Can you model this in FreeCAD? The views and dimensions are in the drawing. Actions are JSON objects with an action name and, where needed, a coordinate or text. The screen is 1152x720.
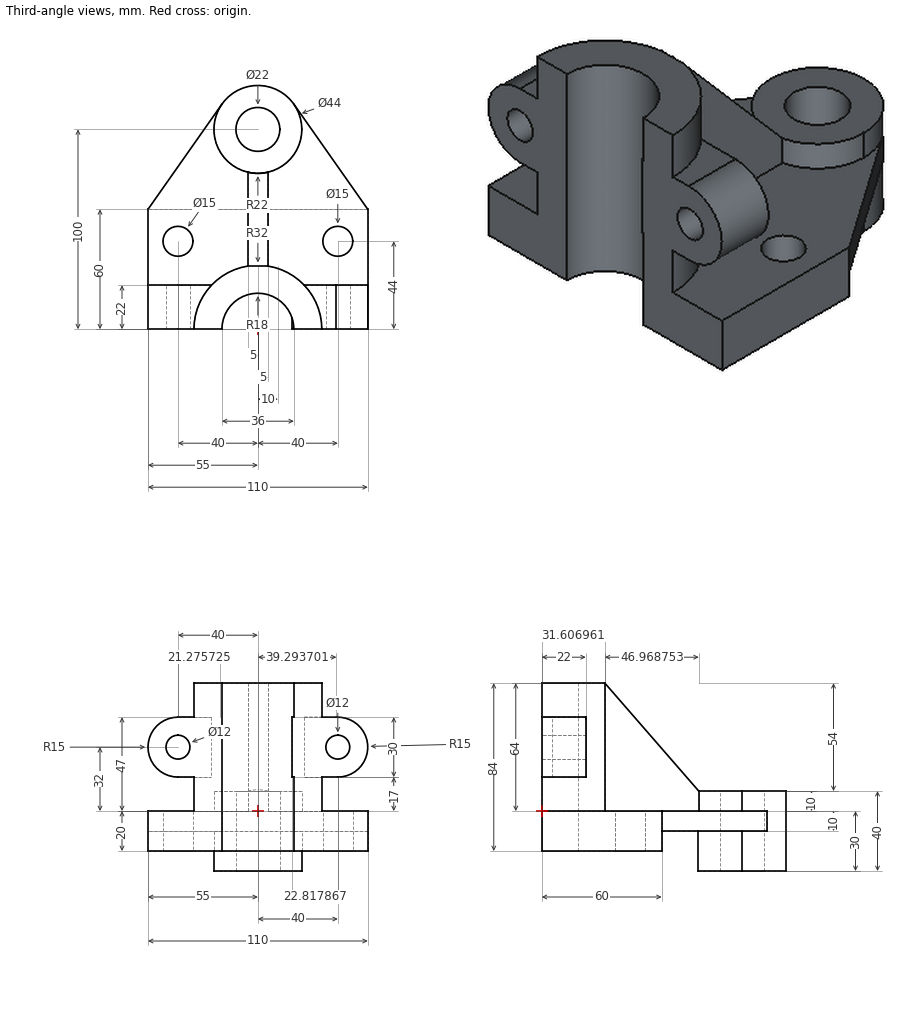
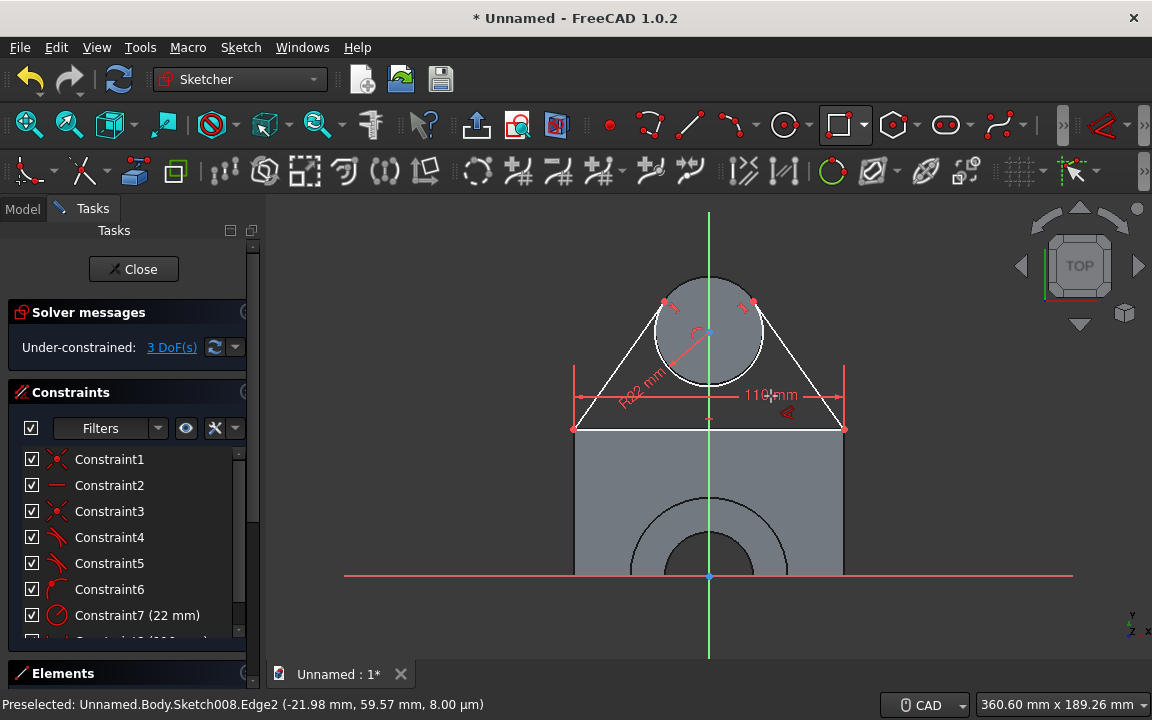
{"action": "left_click", "coordinate": [574, 430]}
{"action": "left_click", "coordinate": [641, 610]}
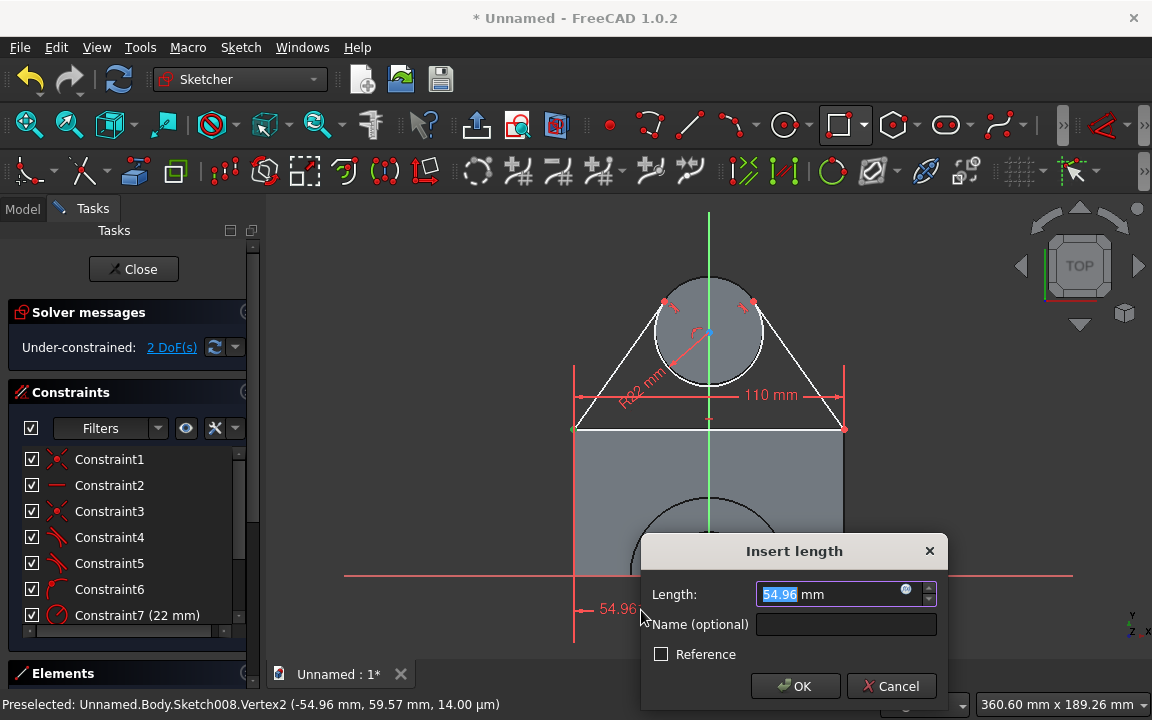
{"action": "type", "text": "55"}
{"action": "key", "text": "Return"}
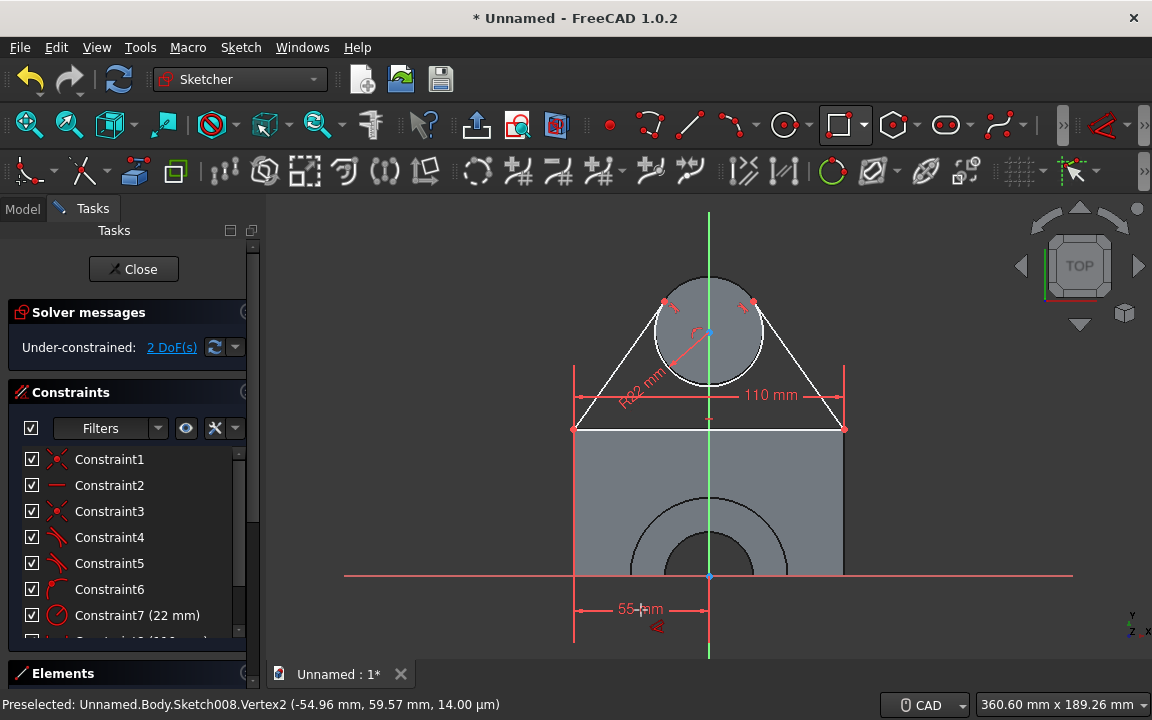
{"action": "left_click", "coordinate": [574, 430]}
{"action": "left_click", "coordinate": [540, 503]}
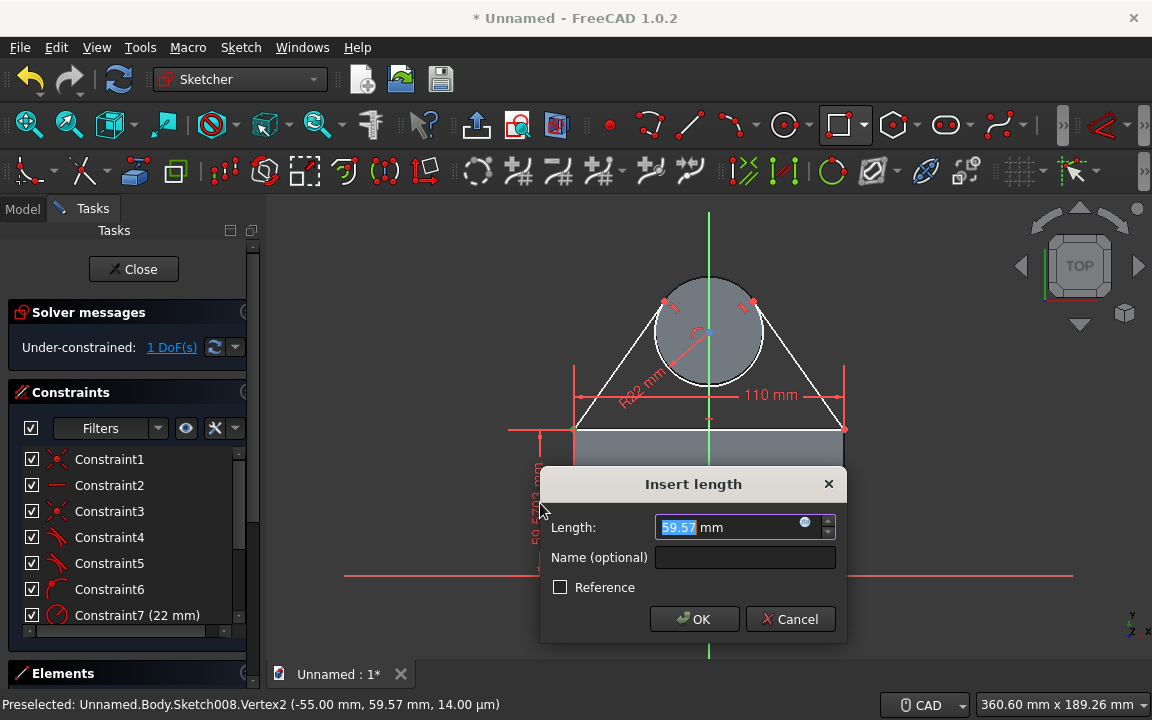
{"action": "type", "text": "60"}
{"action": "key", "text": "Return"}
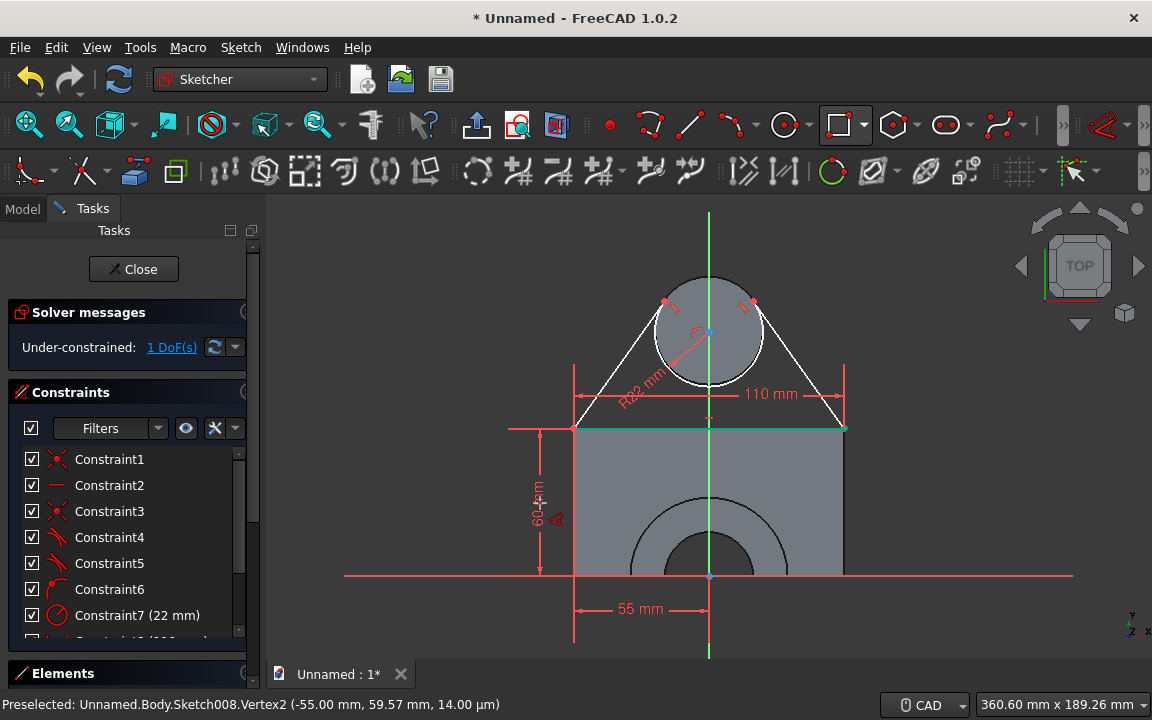
{"action": "left_click", "coordinate": [709, 333]}
{"action": "left_click", "coordinate": [743, 454]}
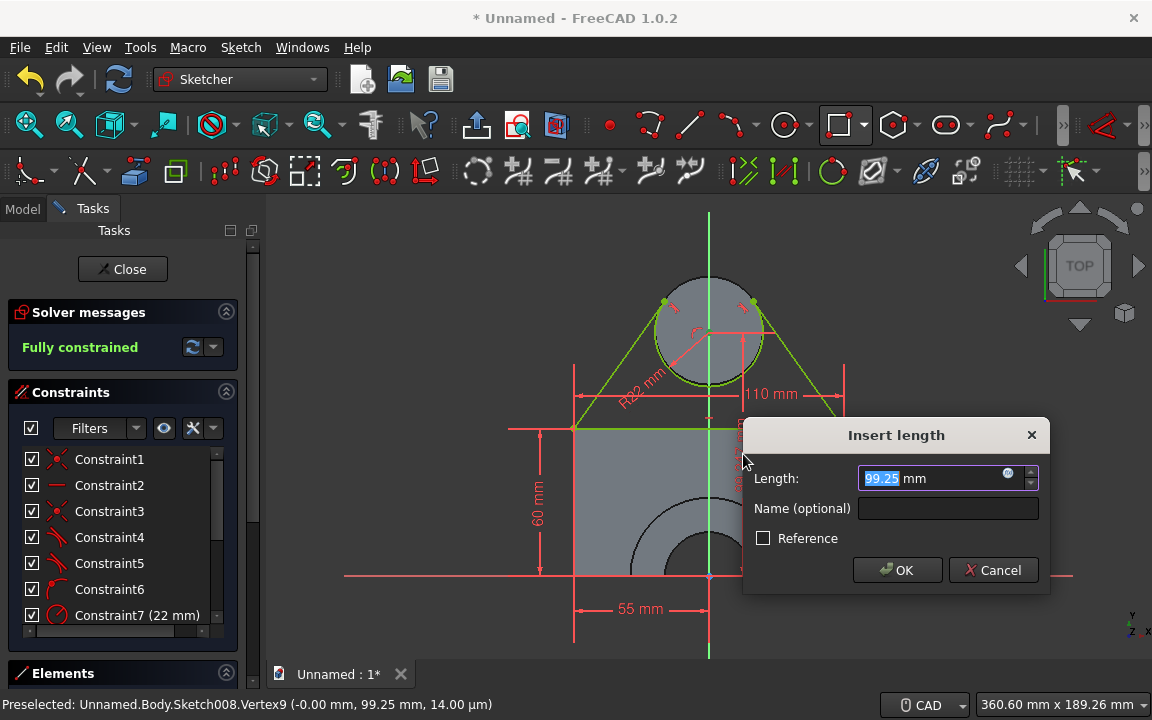
{"action": "type", "text": "100"}
{"action": "key", "text": "Return"}
{"action": "key", "text": "Escape"}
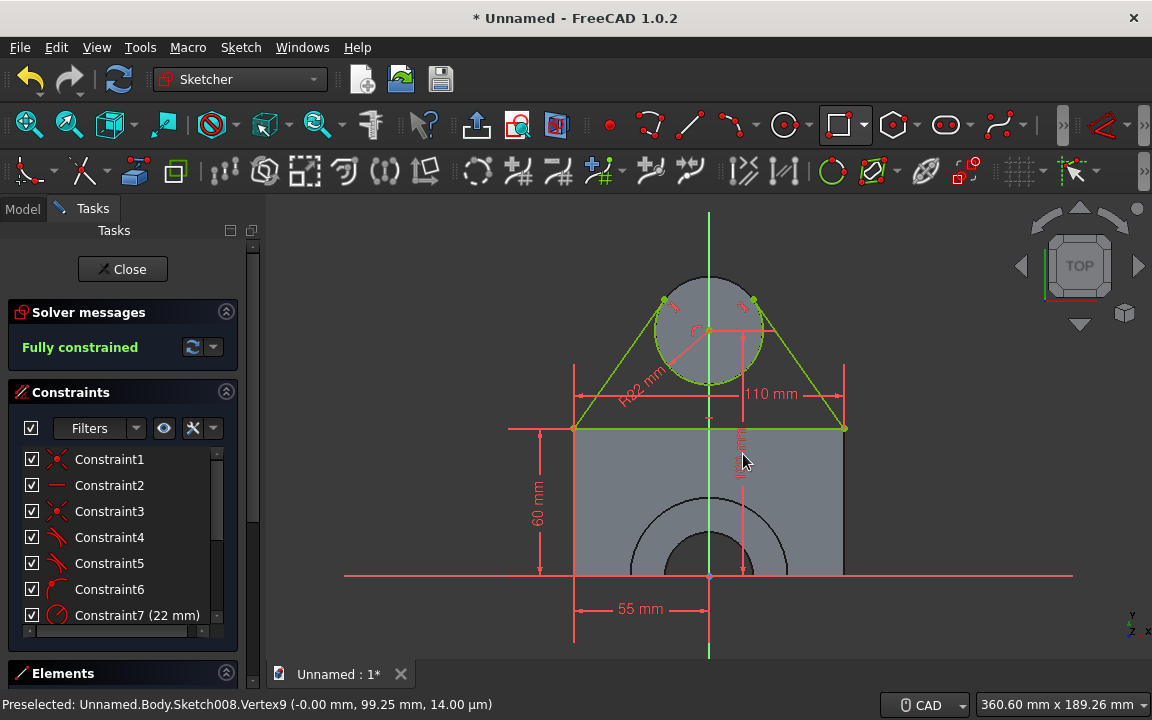
{"action": "left_click", "coordinate": [123, 269]}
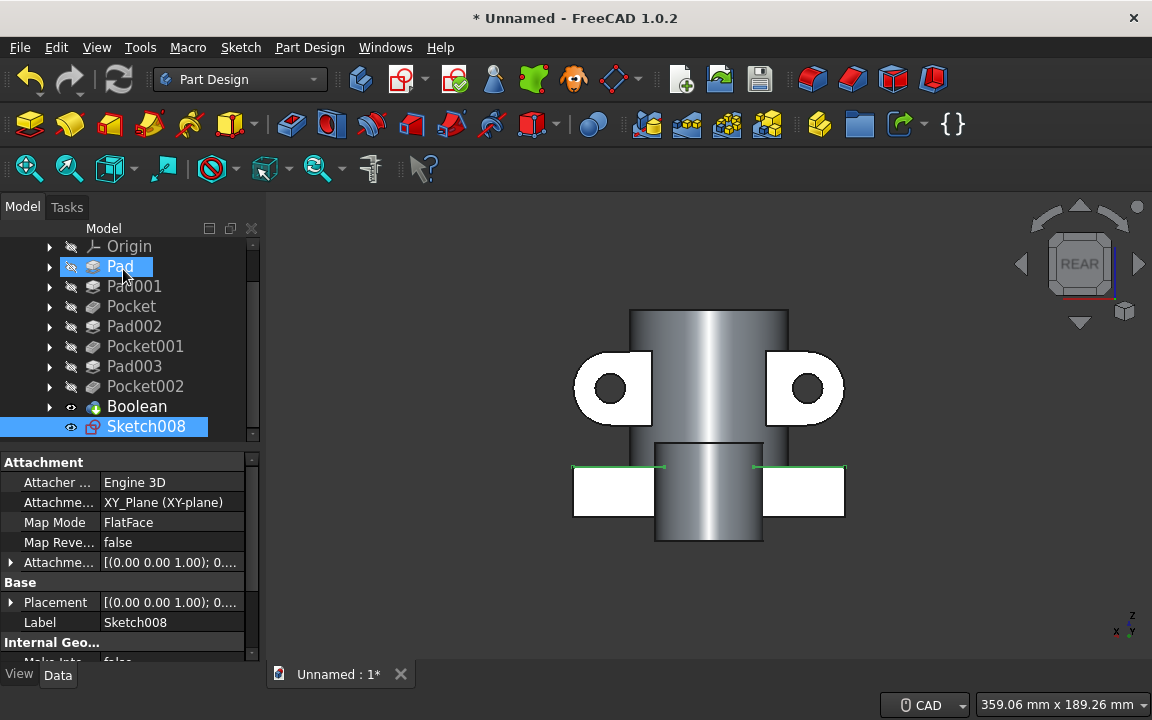
{"action": "left_click", "coordinate": [30, 124]}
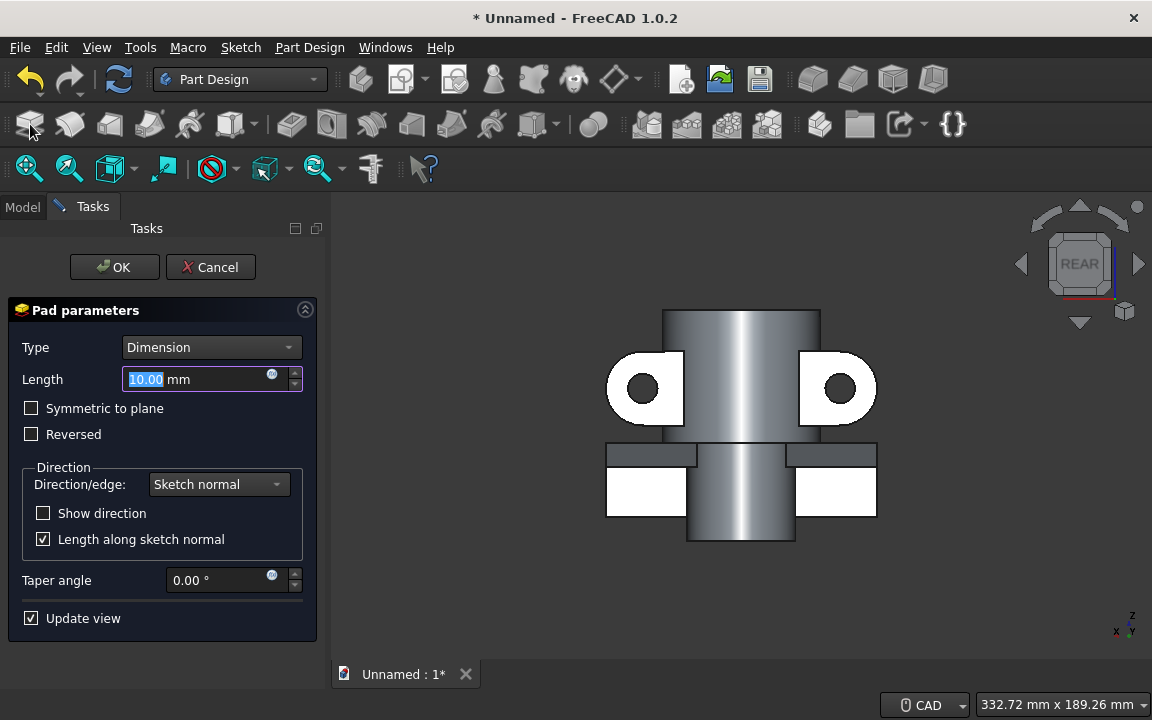
{"action": "type", "text": "10"}
{"action": "key", "text": "Tab"}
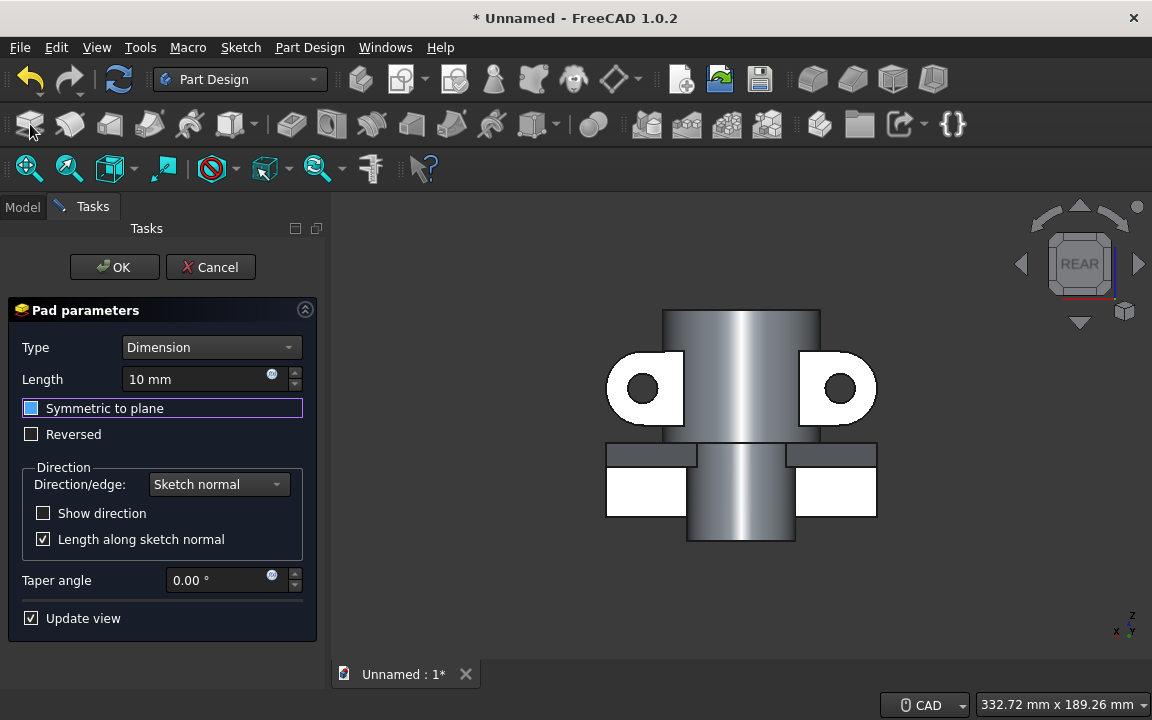
{"action": "left_click", "coordinate": [30, 434]}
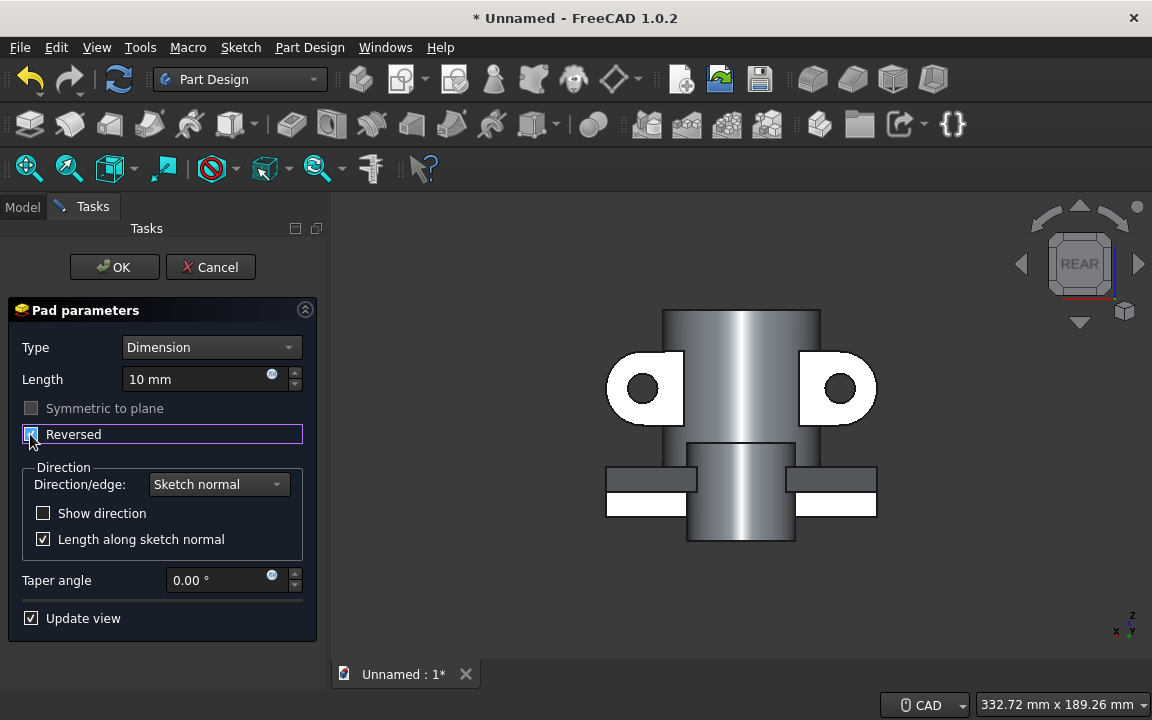
{"action": "left_click", "coordinate": [115, 267]}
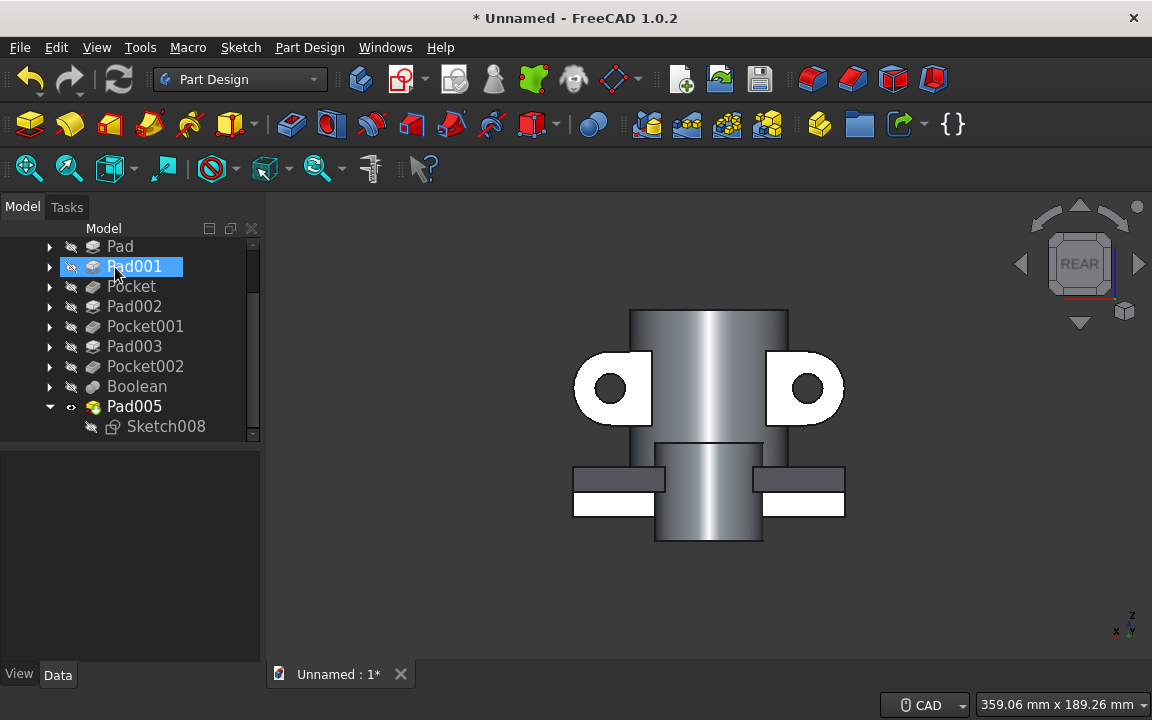
{"action": "key", "text": "0"}